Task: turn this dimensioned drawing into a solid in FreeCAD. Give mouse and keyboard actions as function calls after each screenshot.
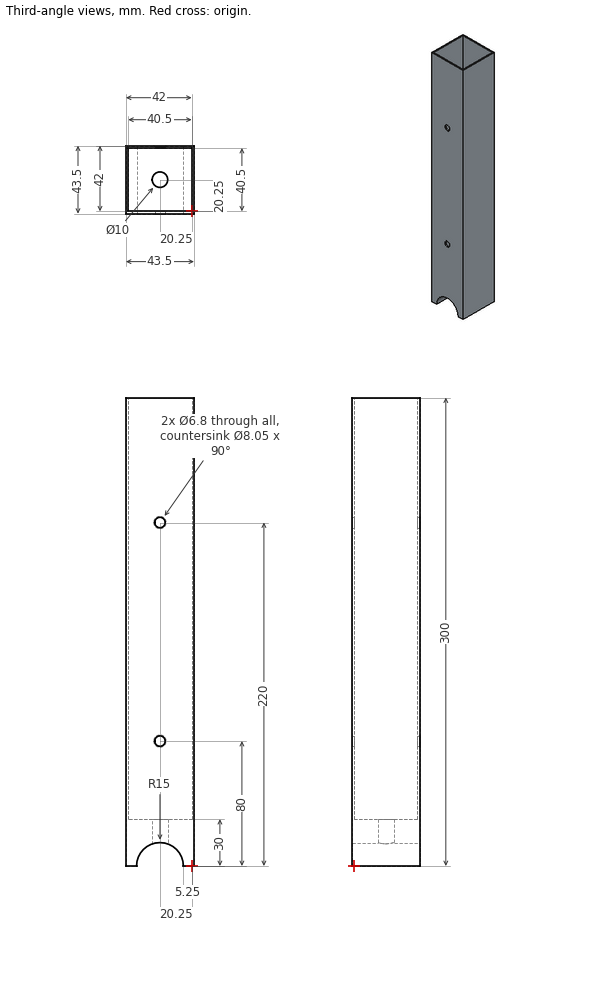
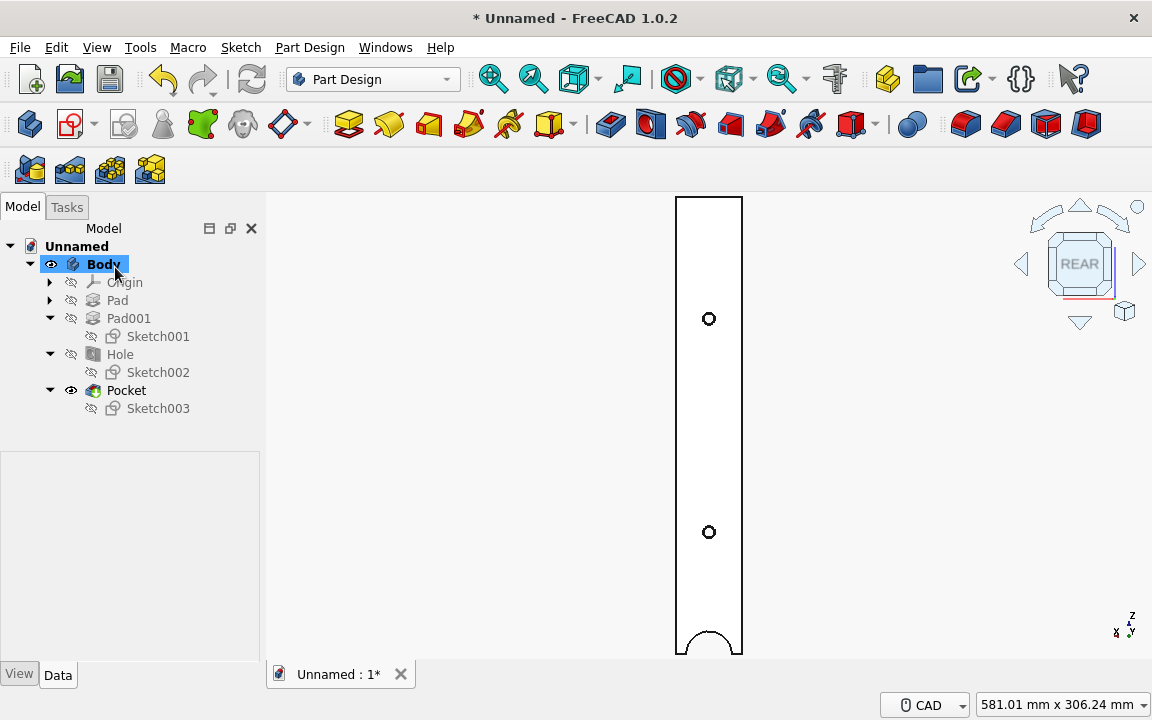
click(70, 124)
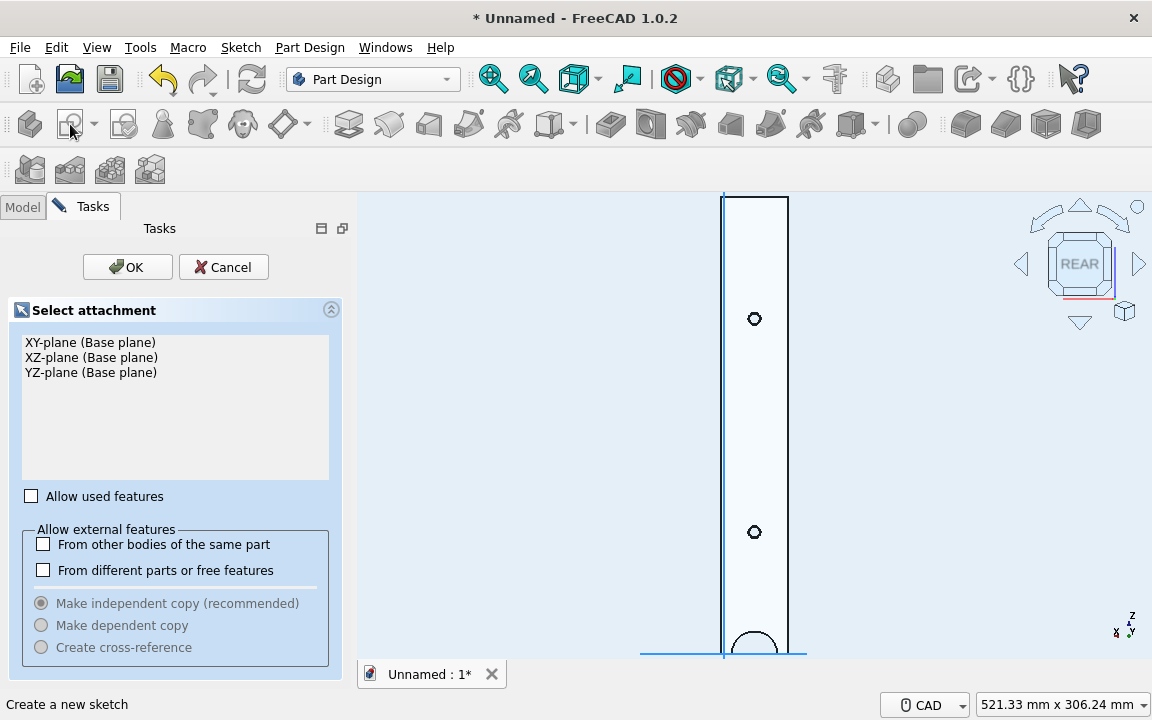
click(82, 342)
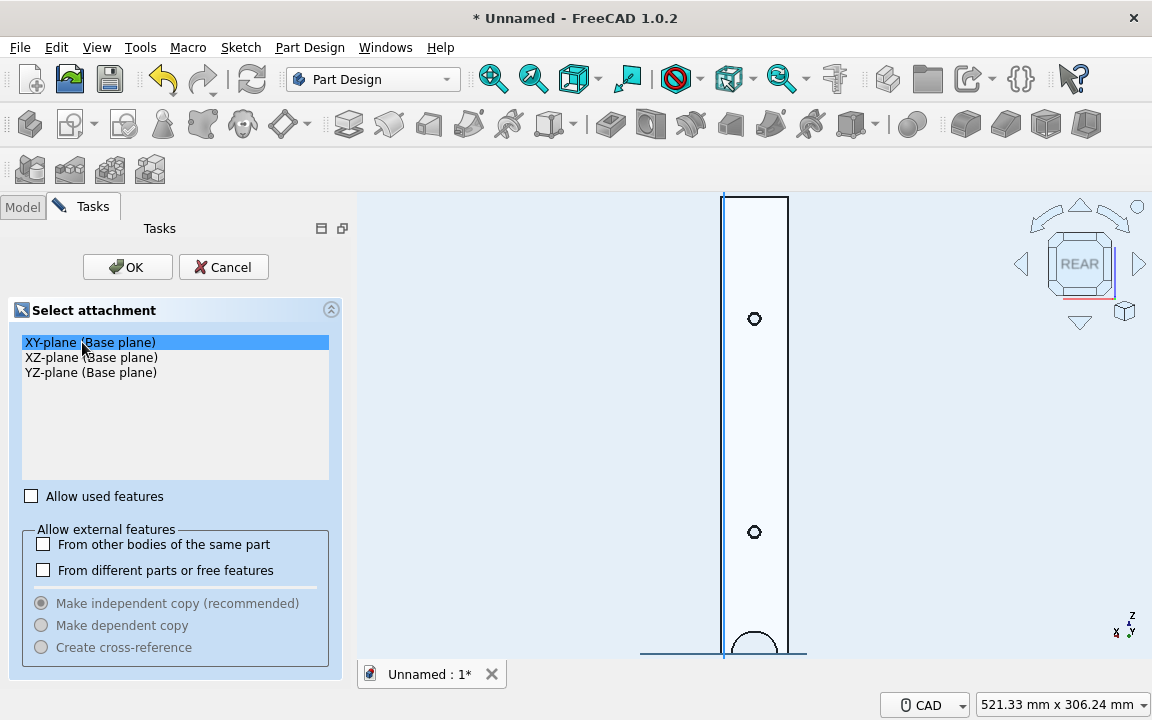
click(128, 267)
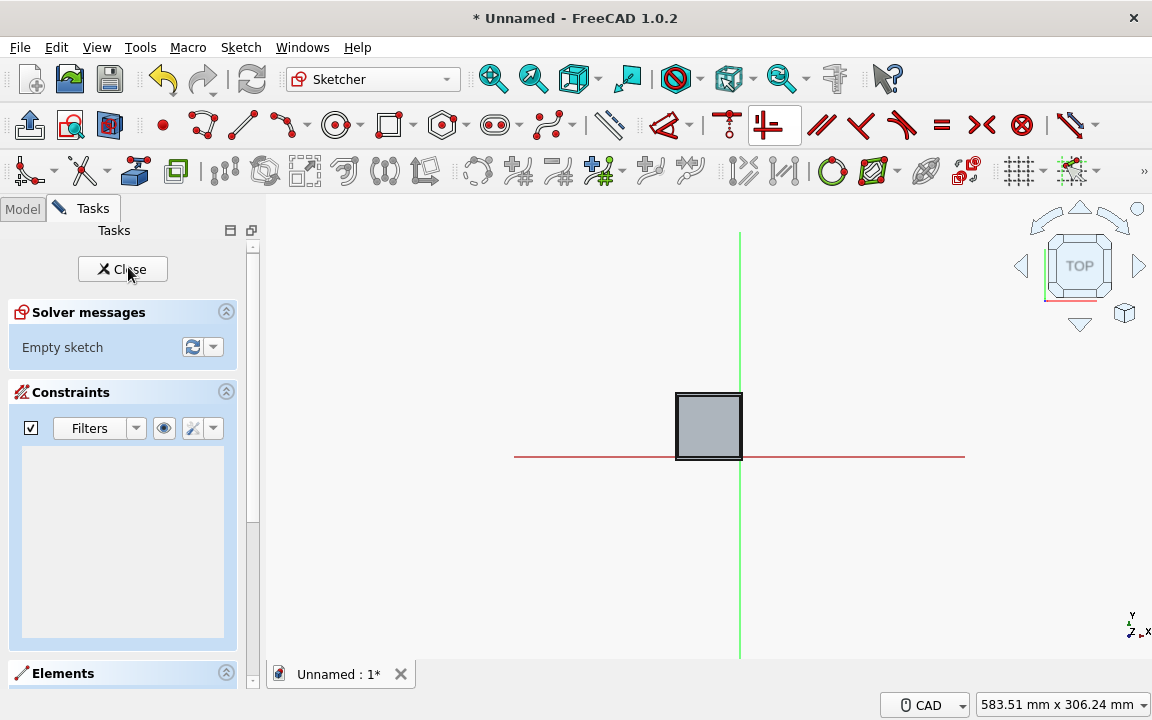
click(110, 126)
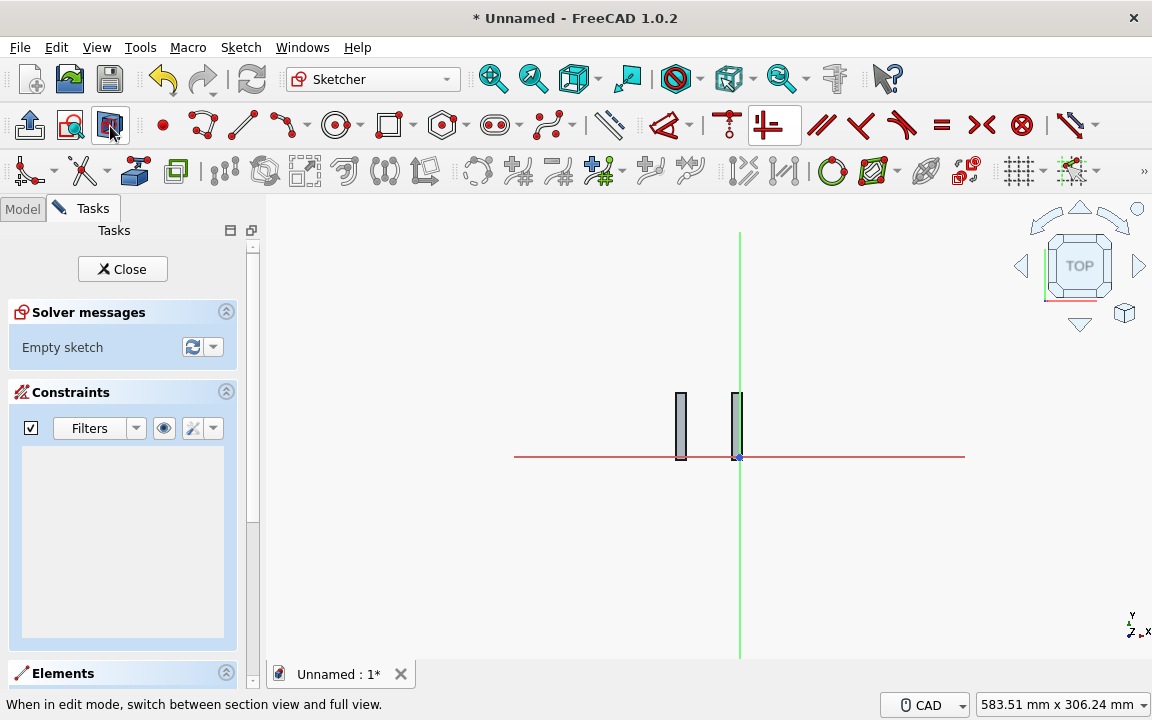
scroll(713, 426, up, 15)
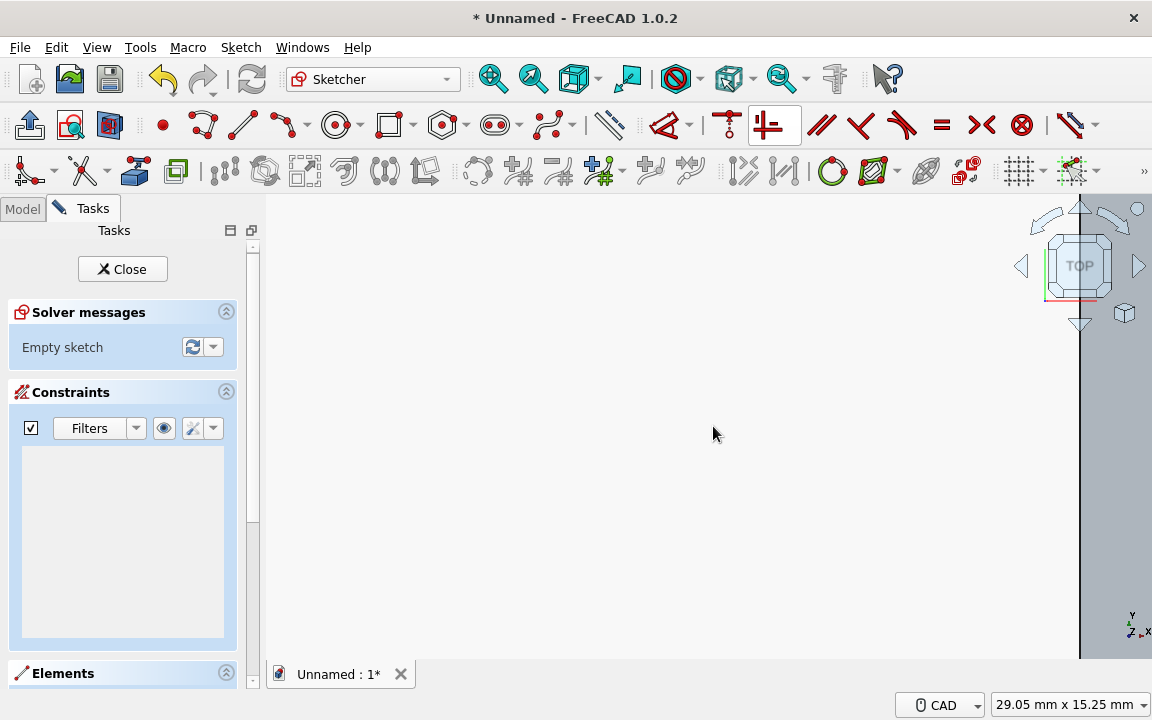
click(336, 126)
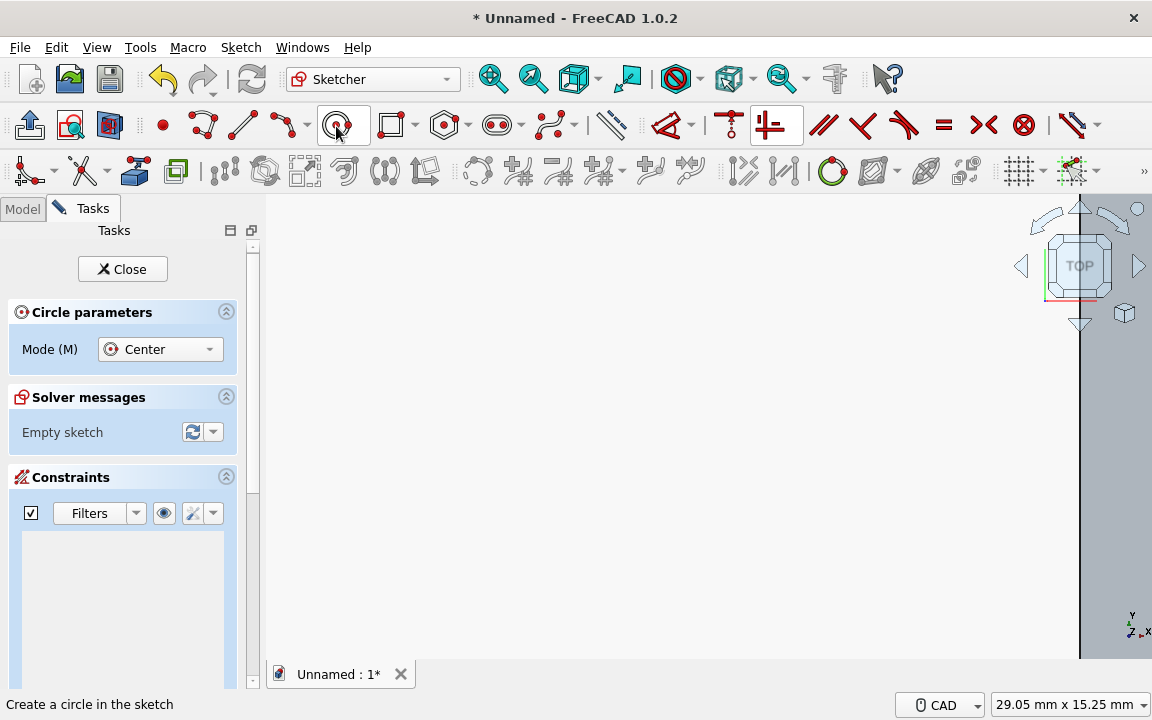
click(623, 426)
click(731, 319)
key(Escape)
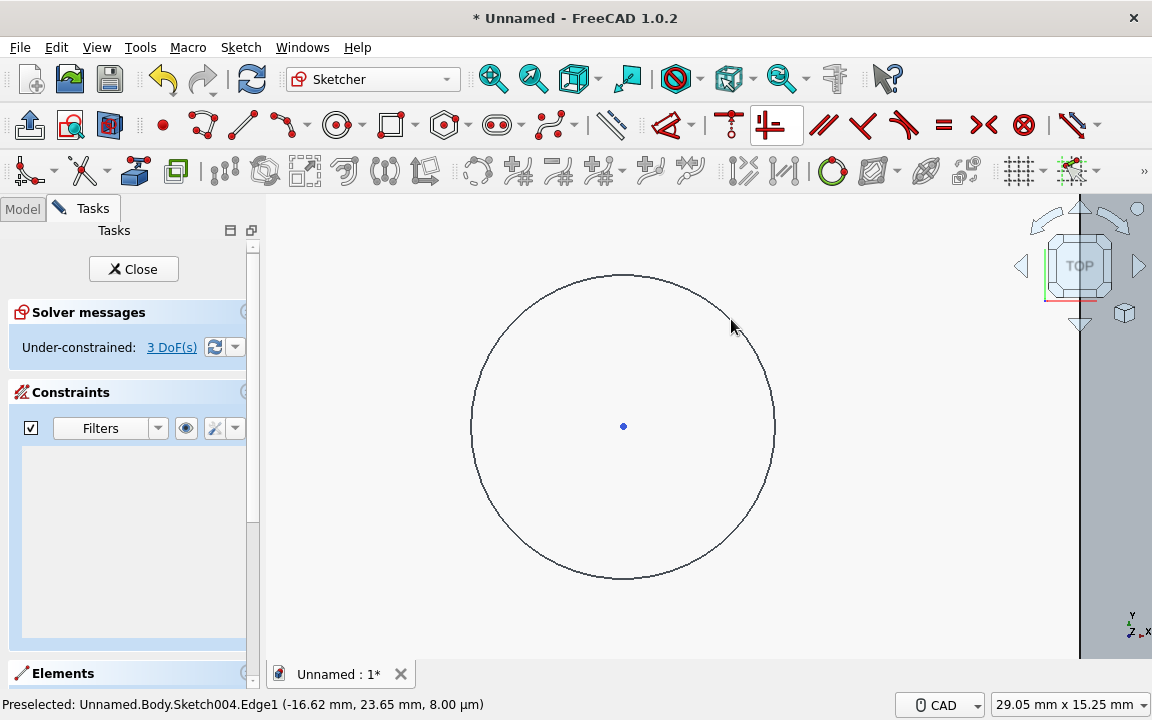
click(666, 126)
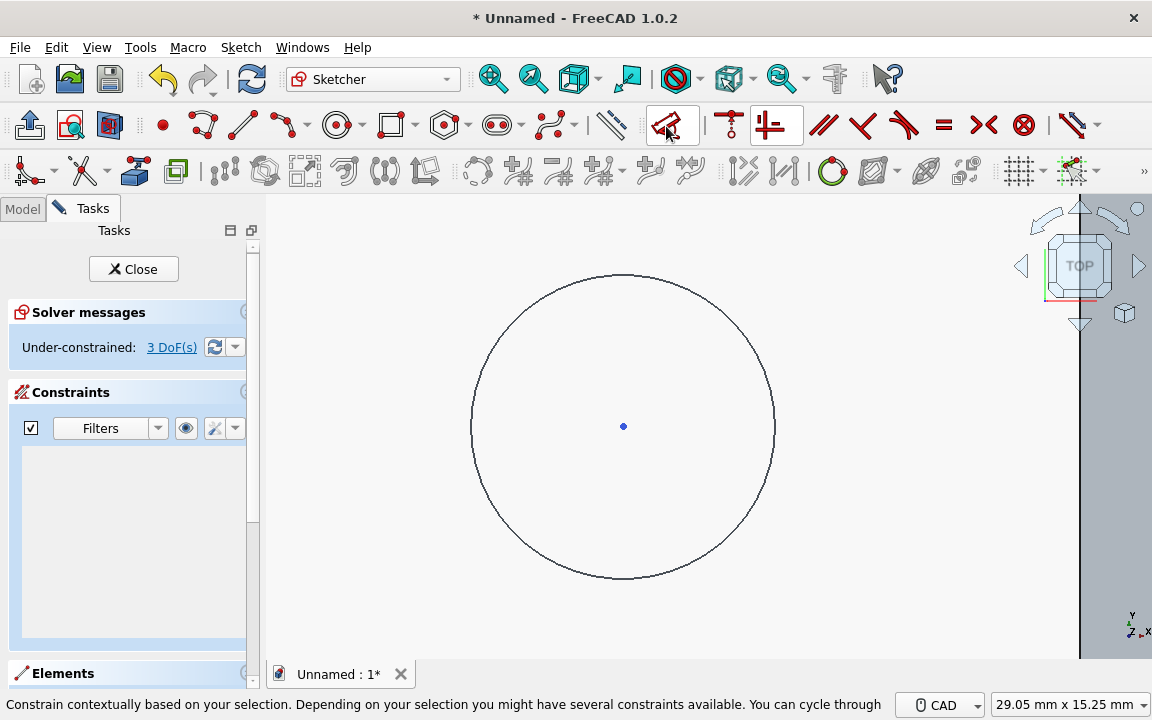
click(730, 319)
click(753, 296)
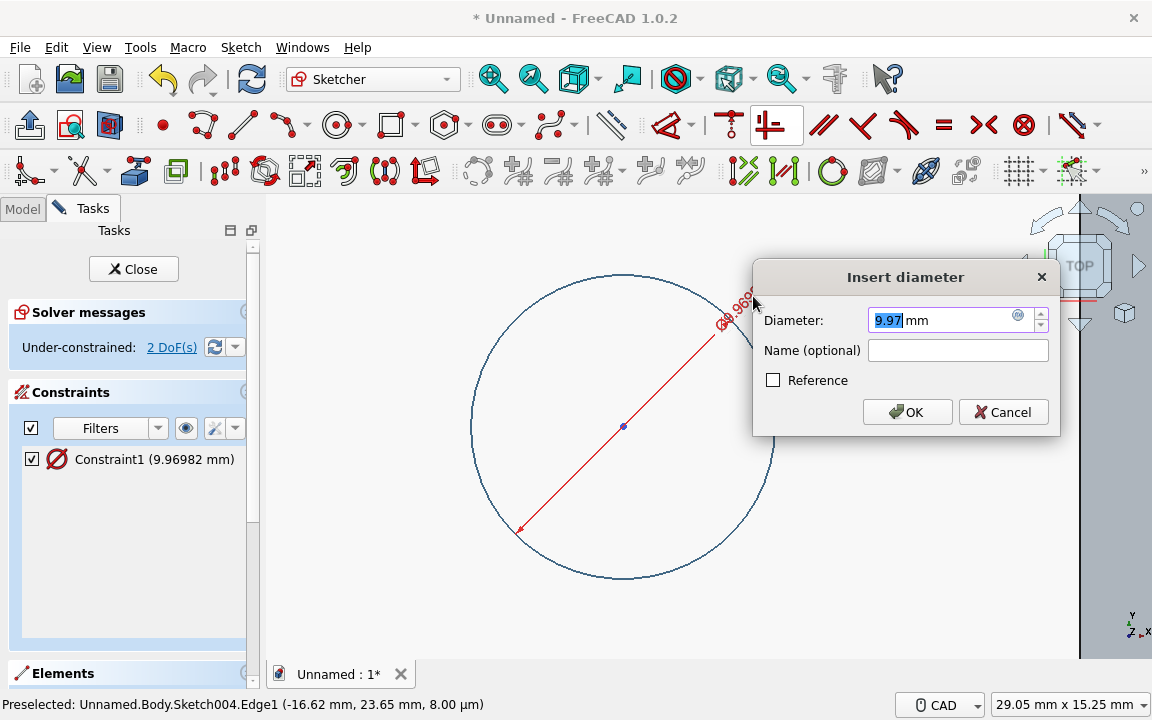
text(10)
key(Return)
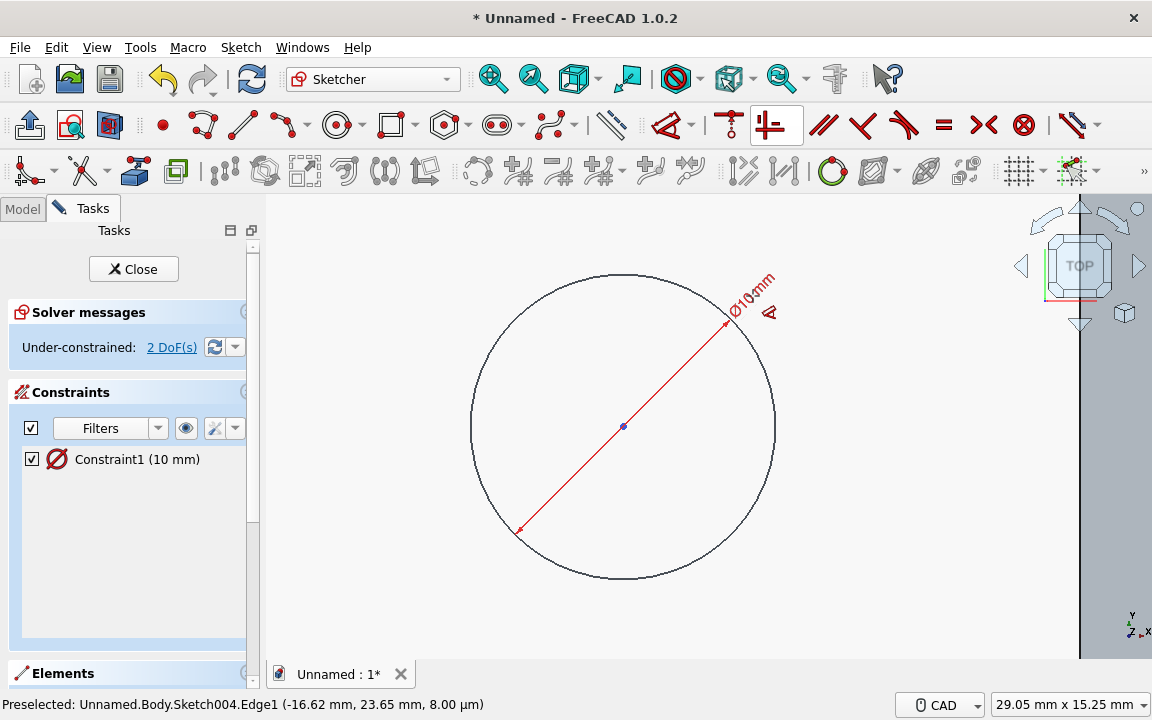
click(623, 427)
click(805, 393)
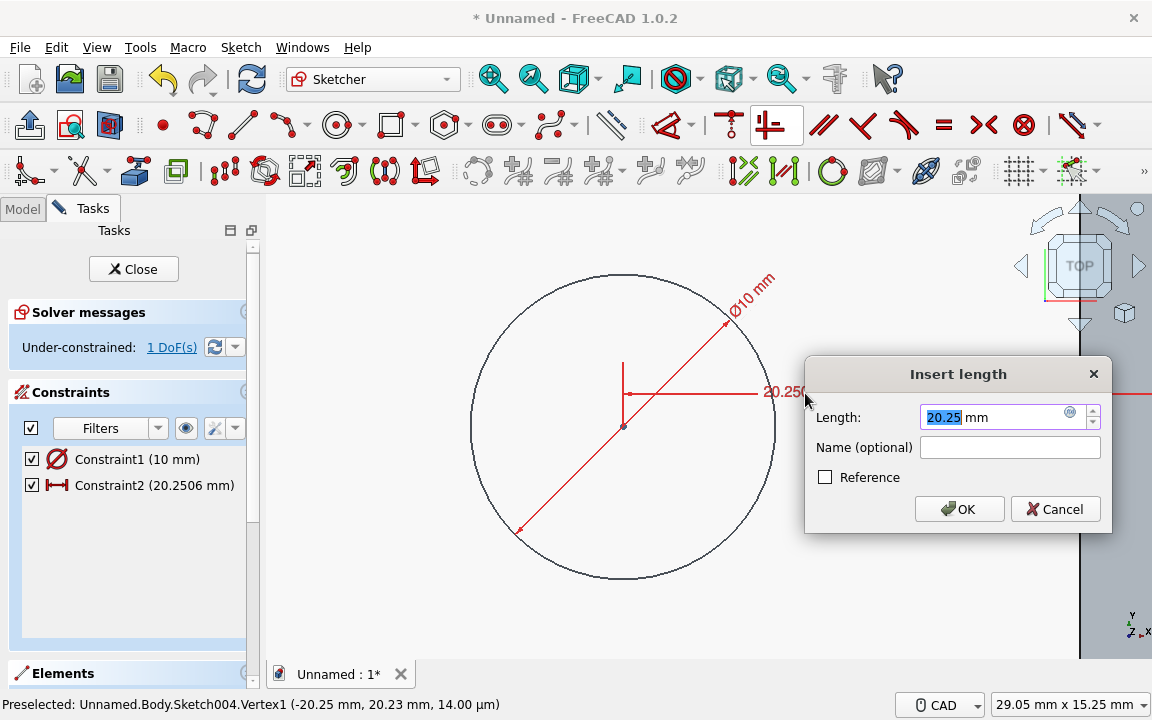
text(20.25)
key(Return)